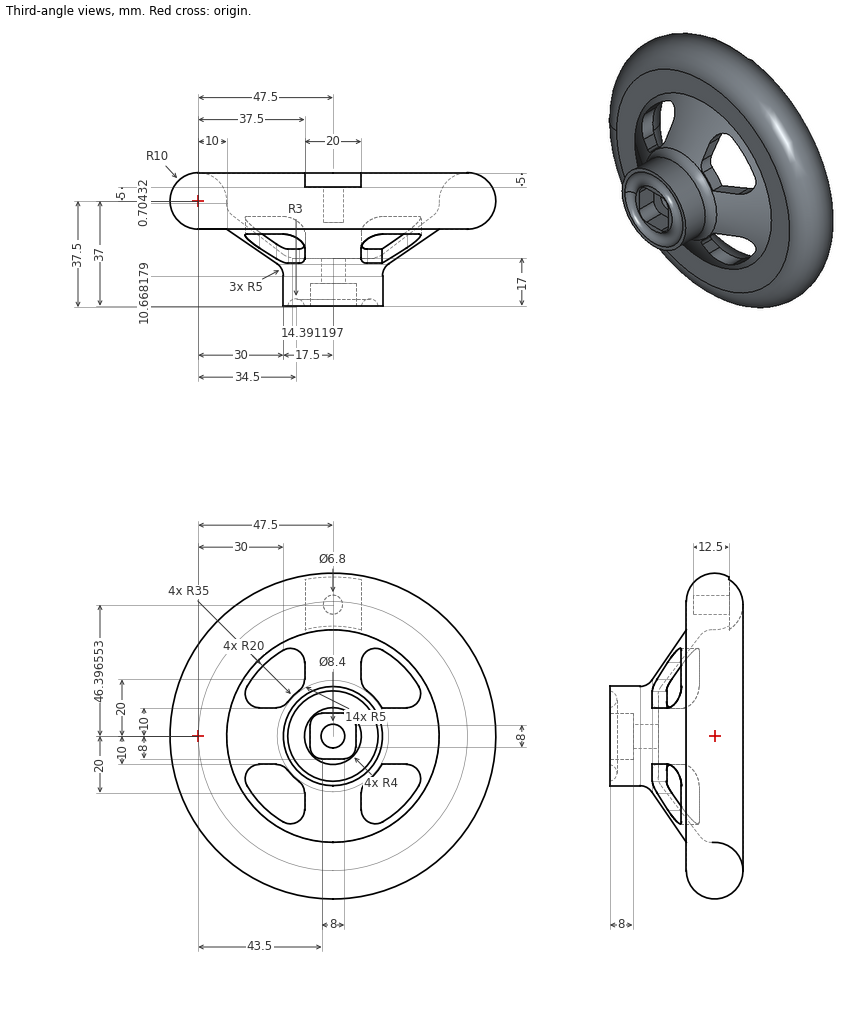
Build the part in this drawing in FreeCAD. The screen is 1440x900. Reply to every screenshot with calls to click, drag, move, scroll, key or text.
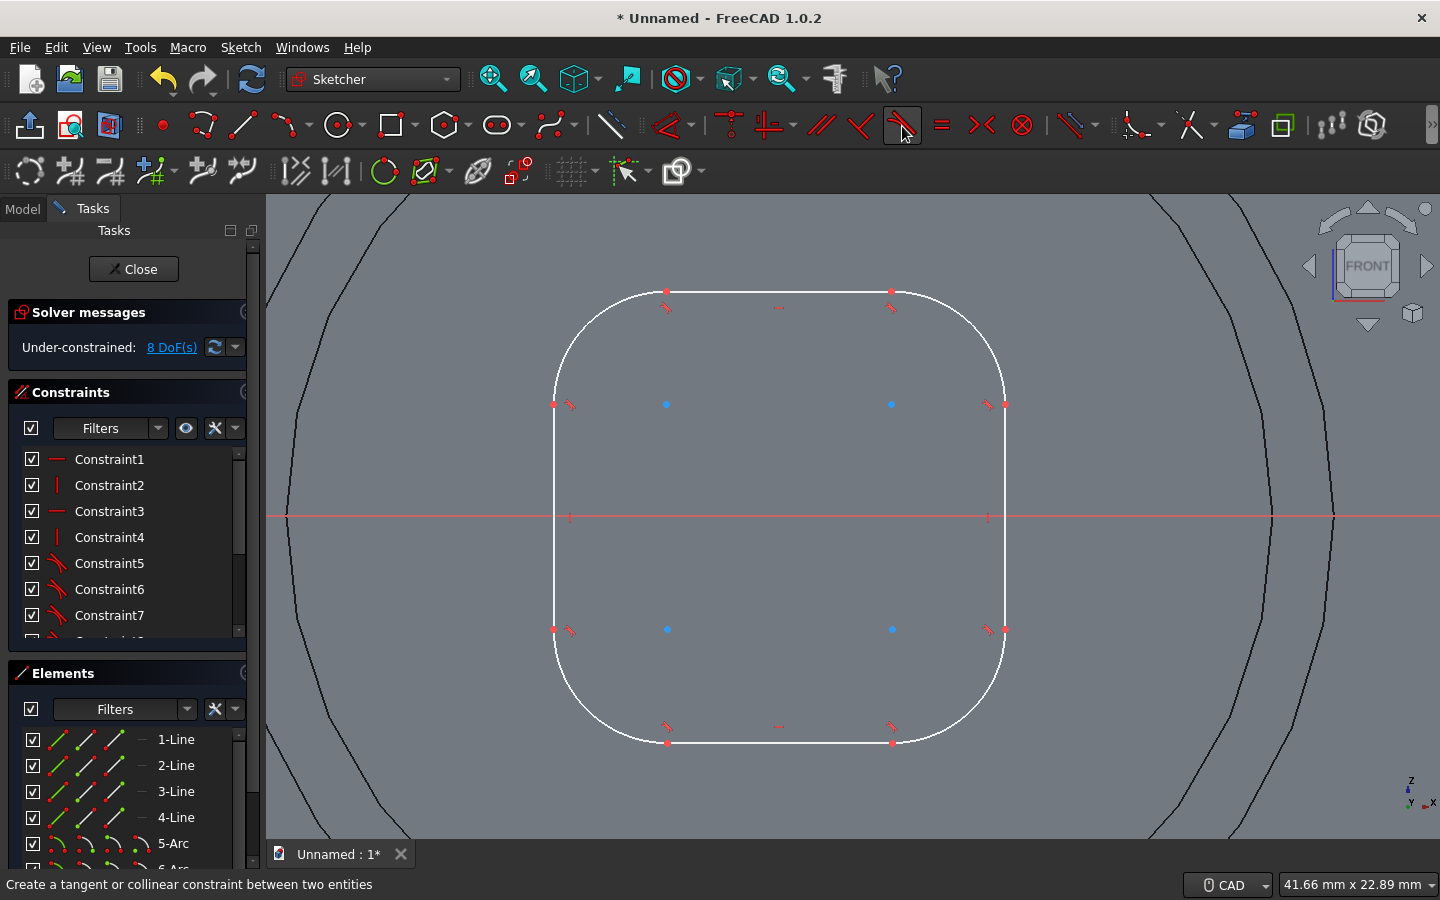
click(943, 731)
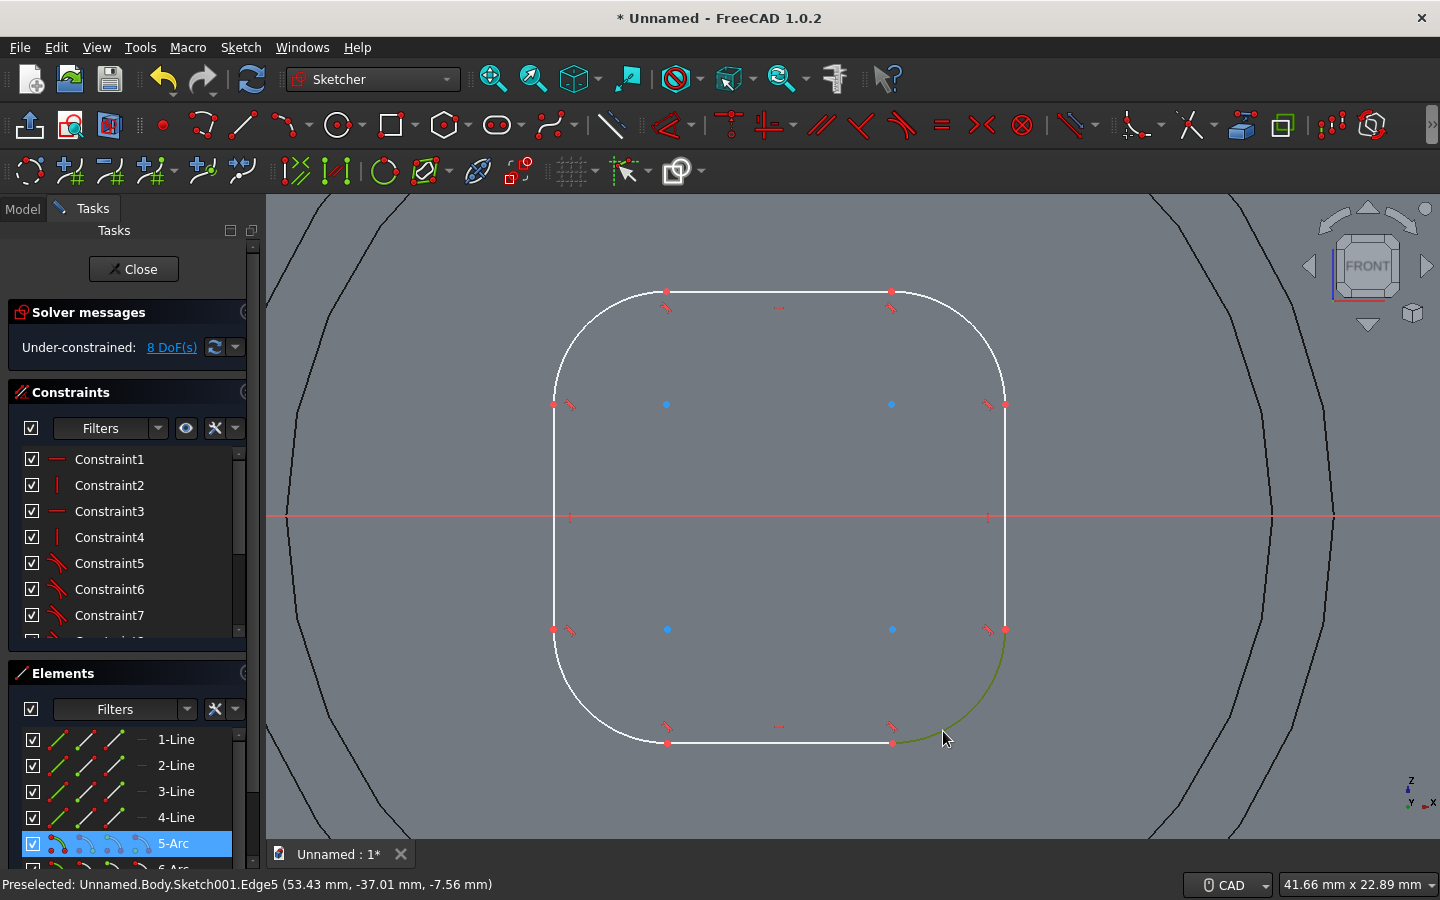
click(993, 353)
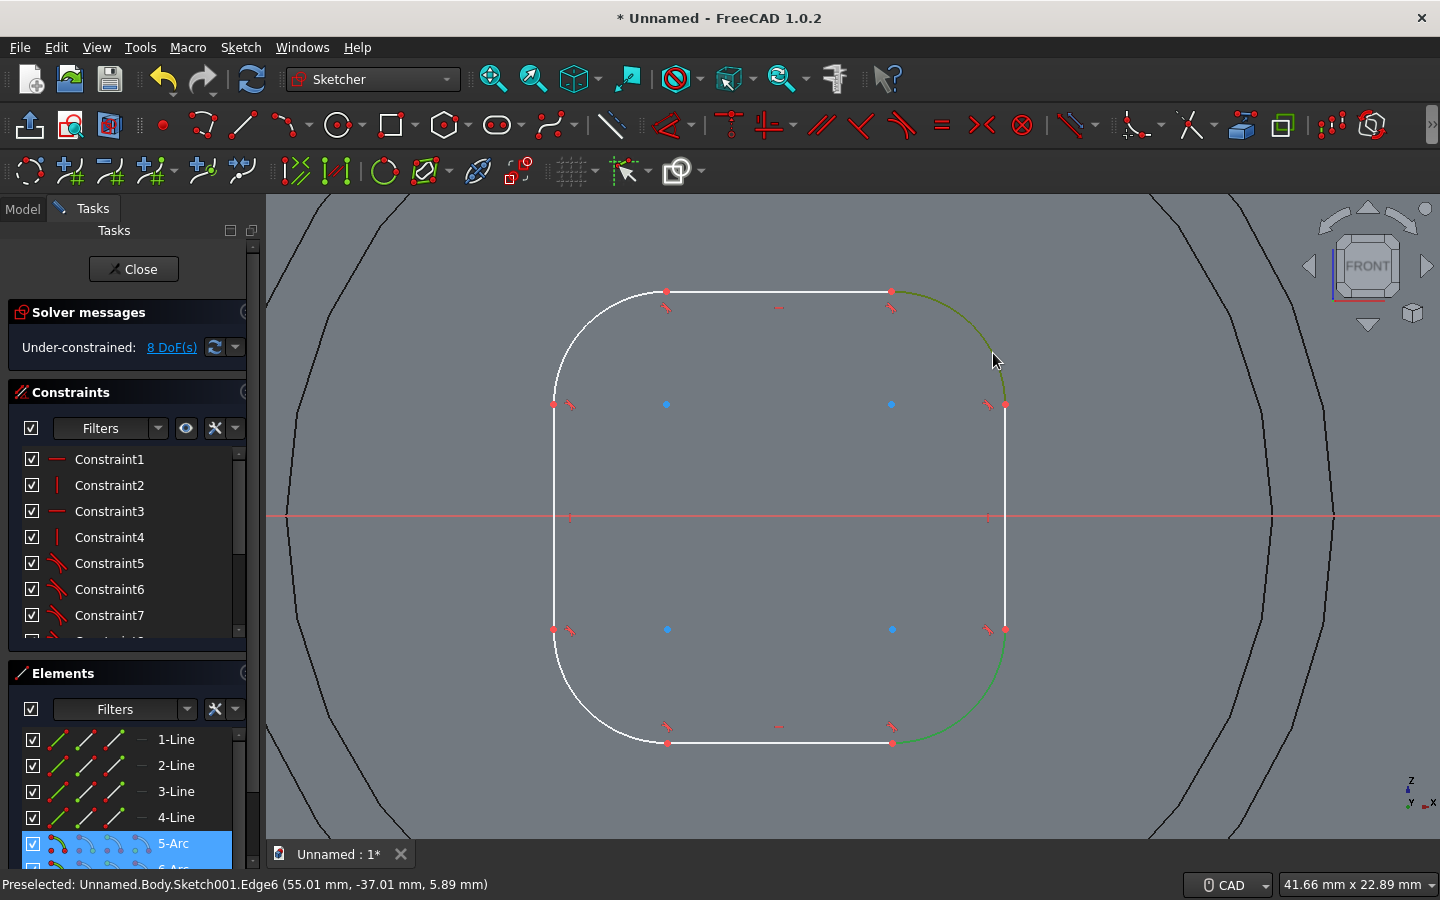
click(616, 304)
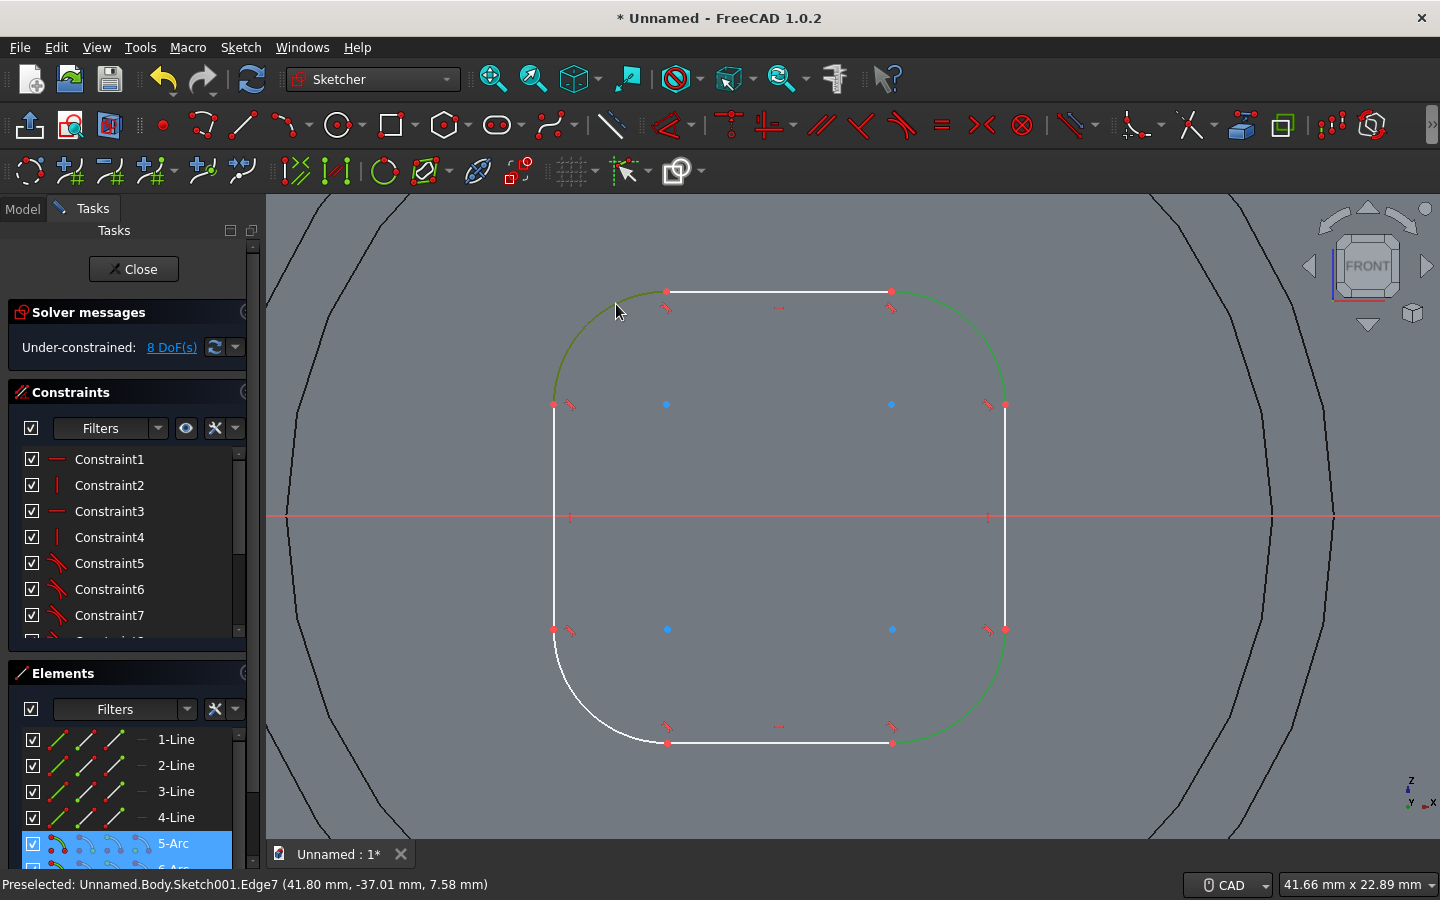
click(566, 681)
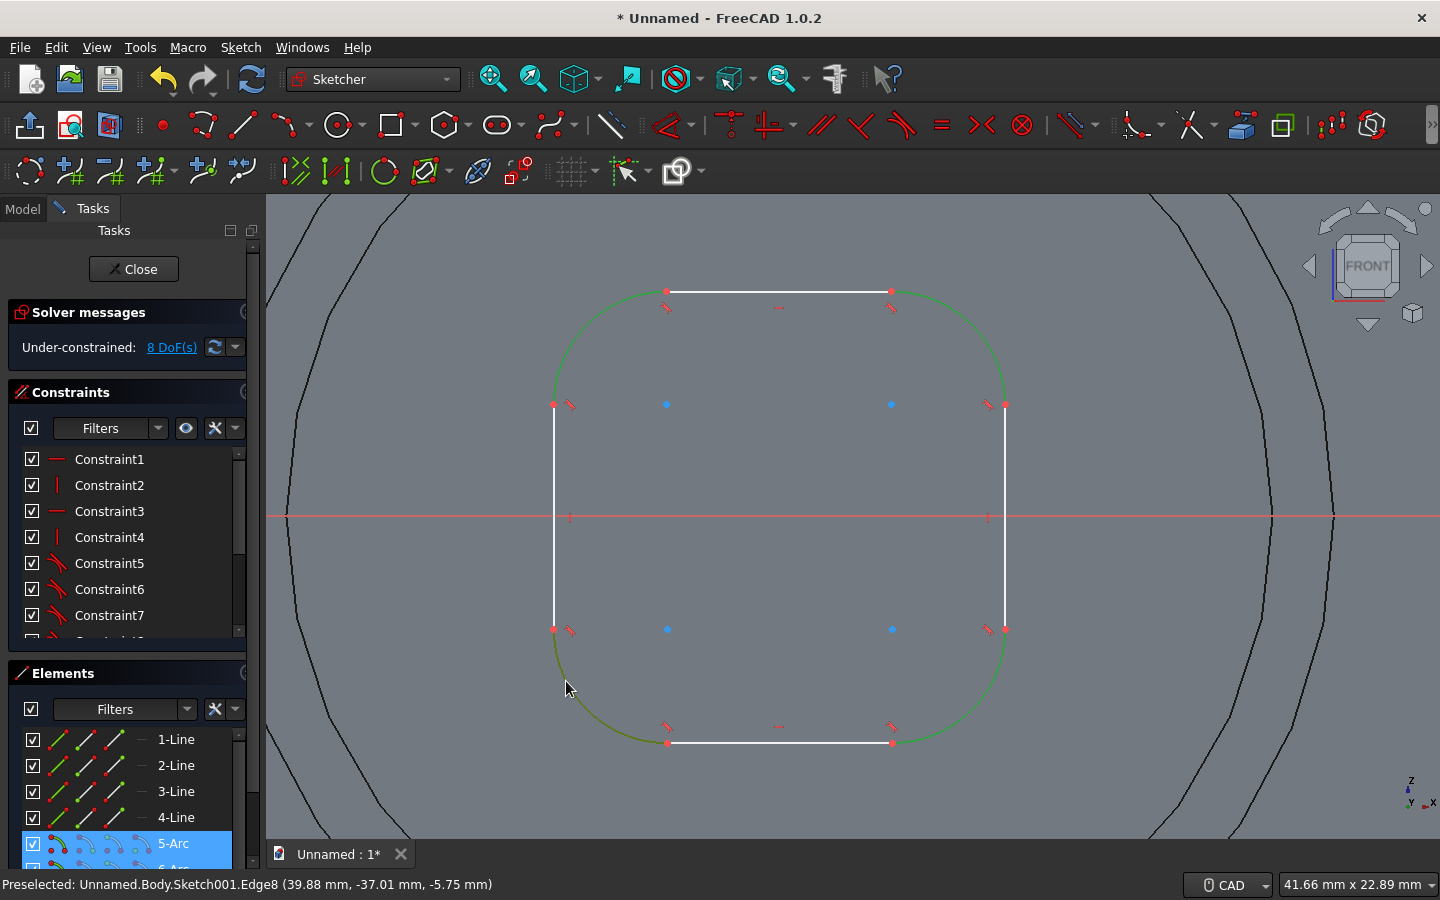
click(942, 126)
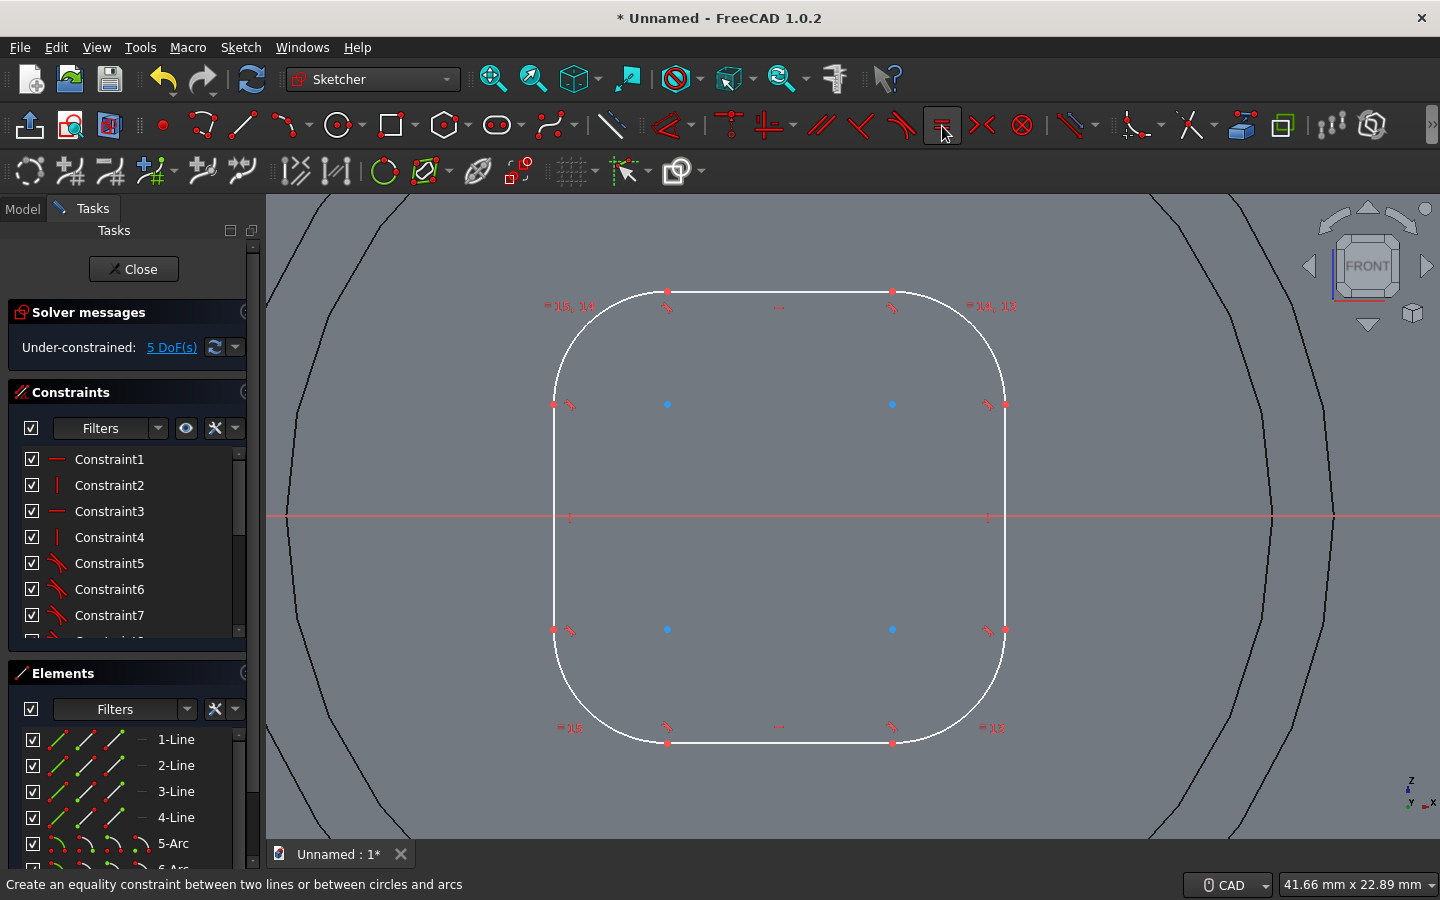
click(666, 126)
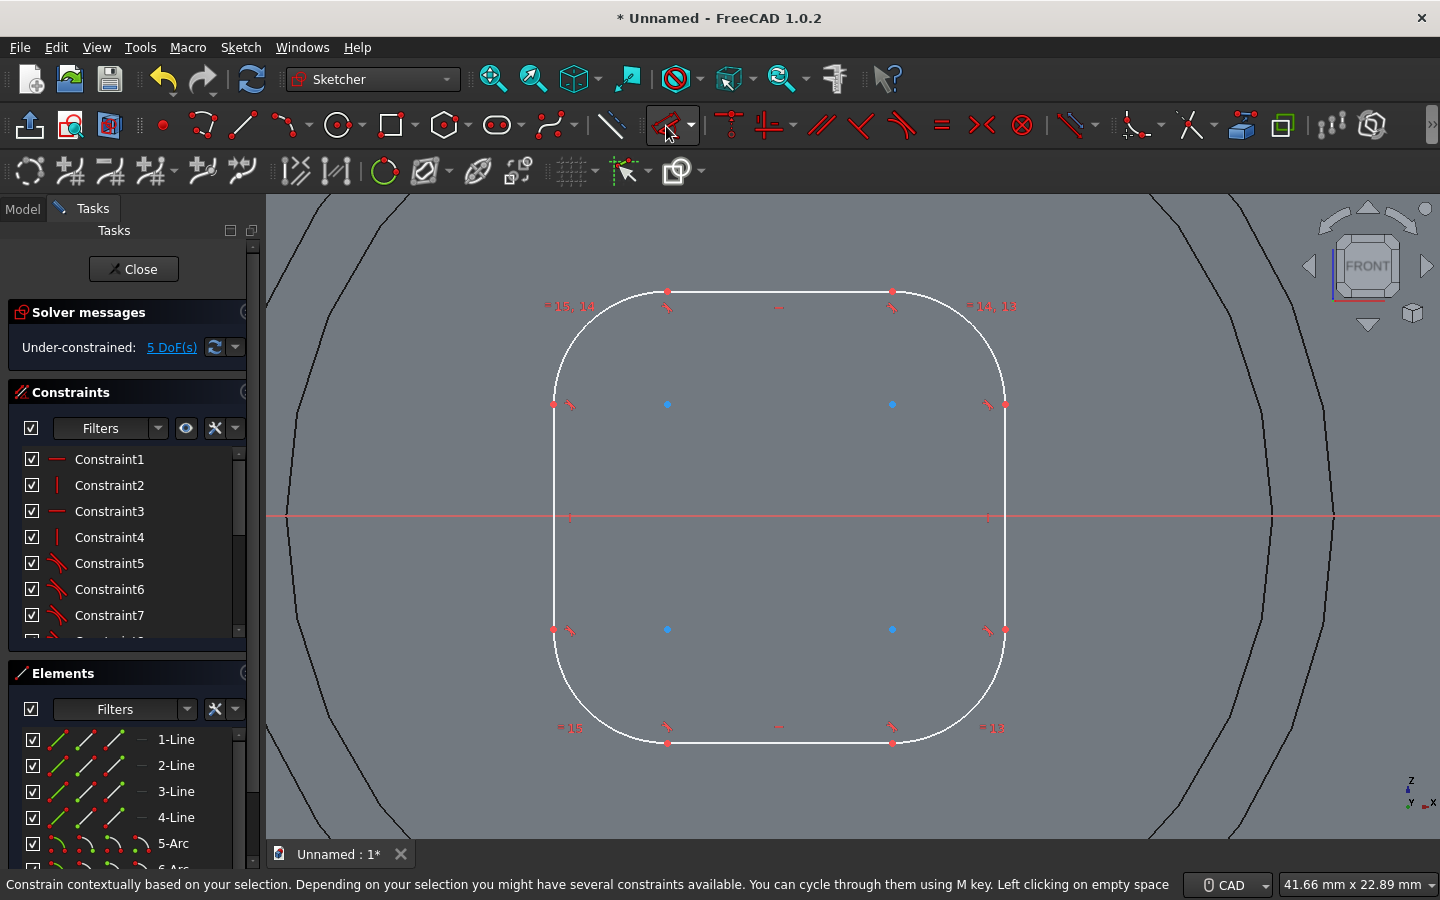
click(943, 731)
click(957, 760)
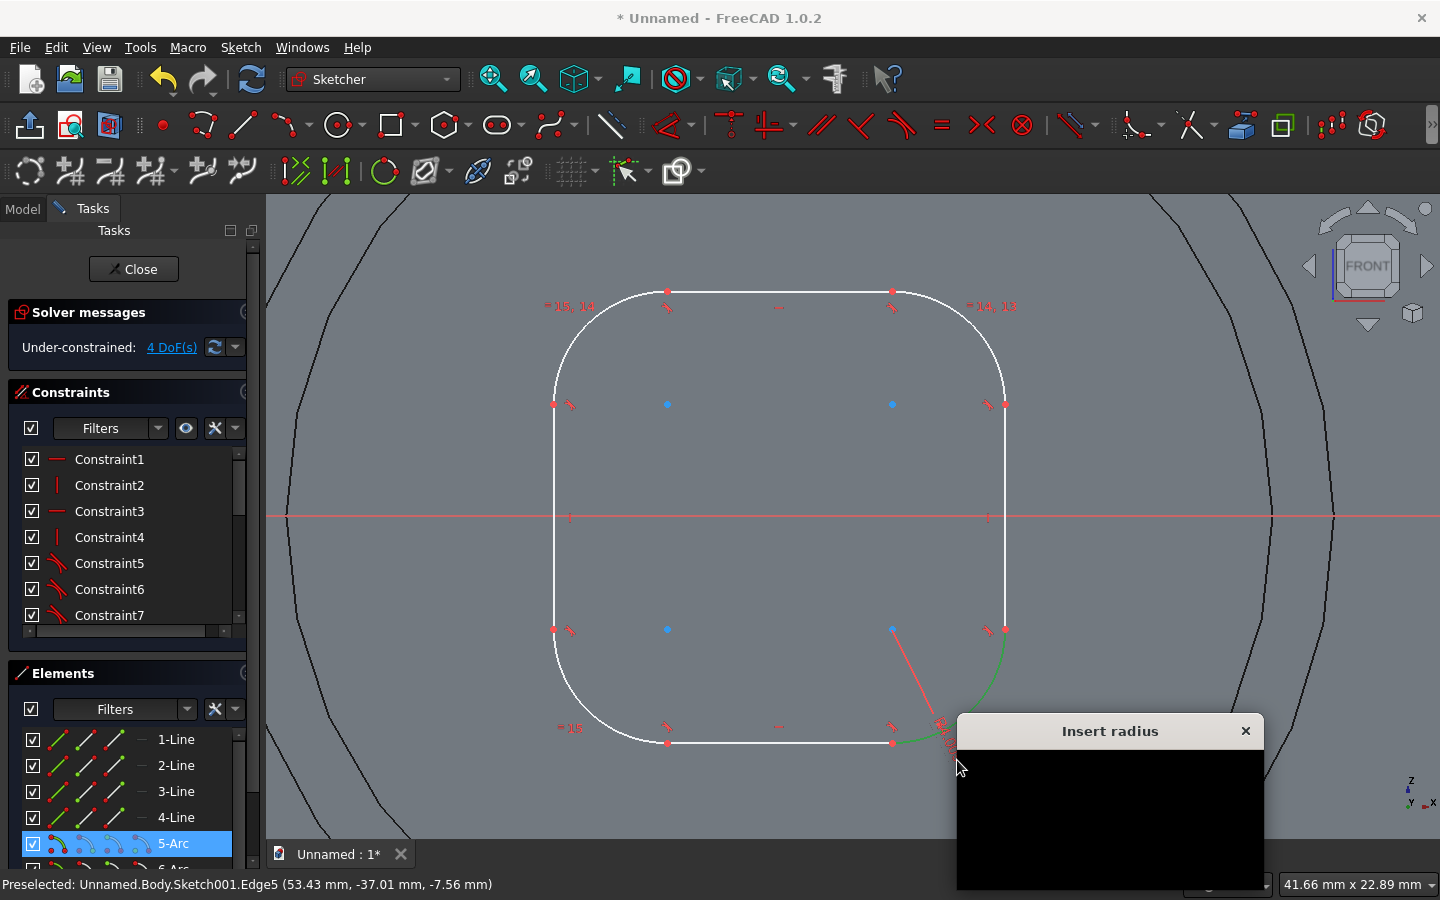
text(4)
key(Return)